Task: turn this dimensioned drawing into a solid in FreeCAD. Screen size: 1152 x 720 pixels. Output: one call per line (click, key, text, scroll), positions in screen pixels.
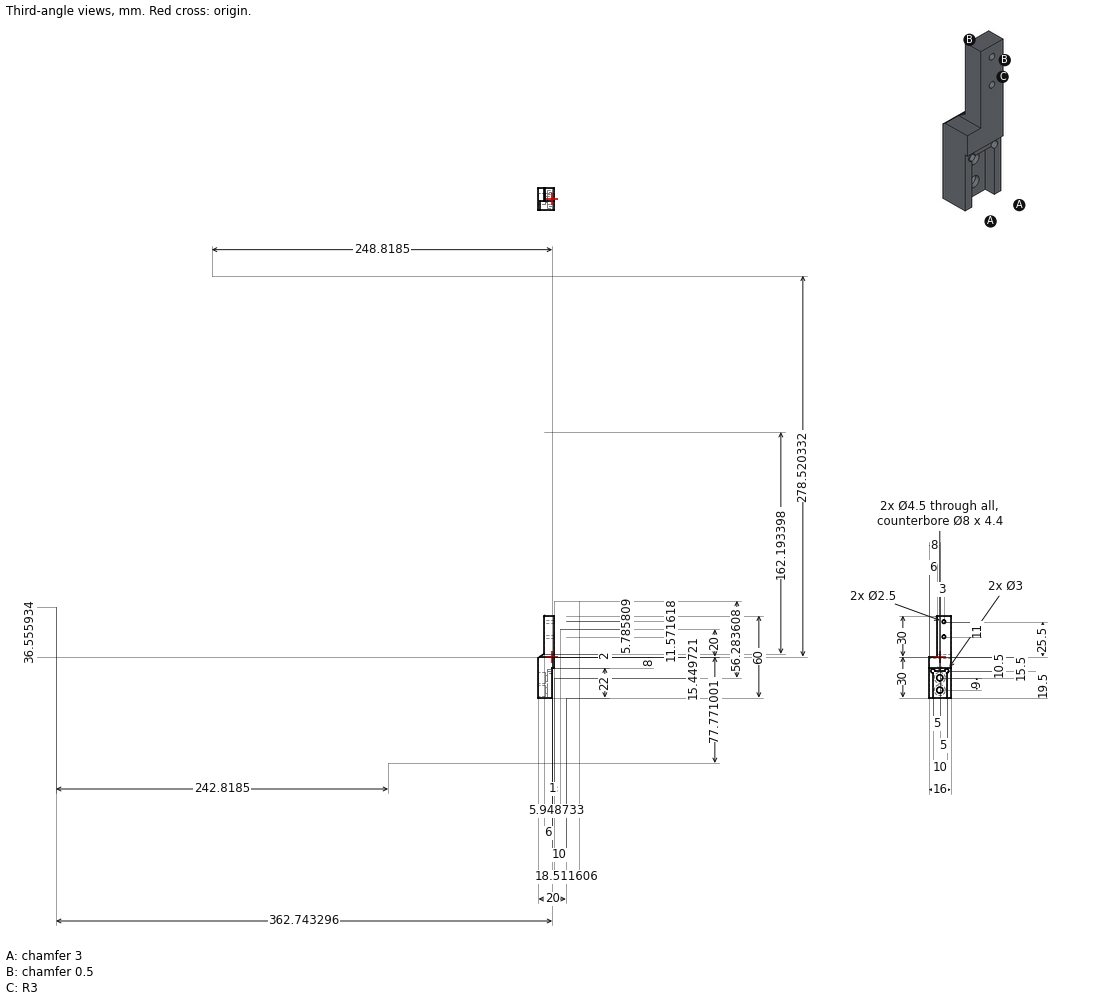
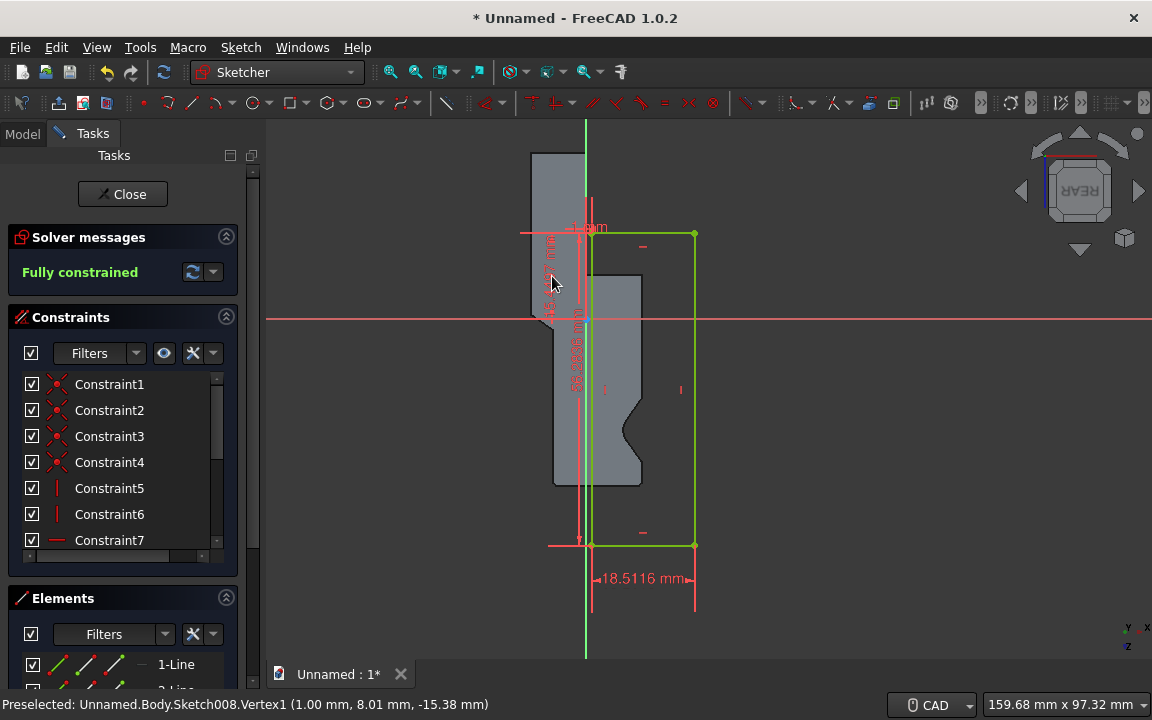
click(123, 194)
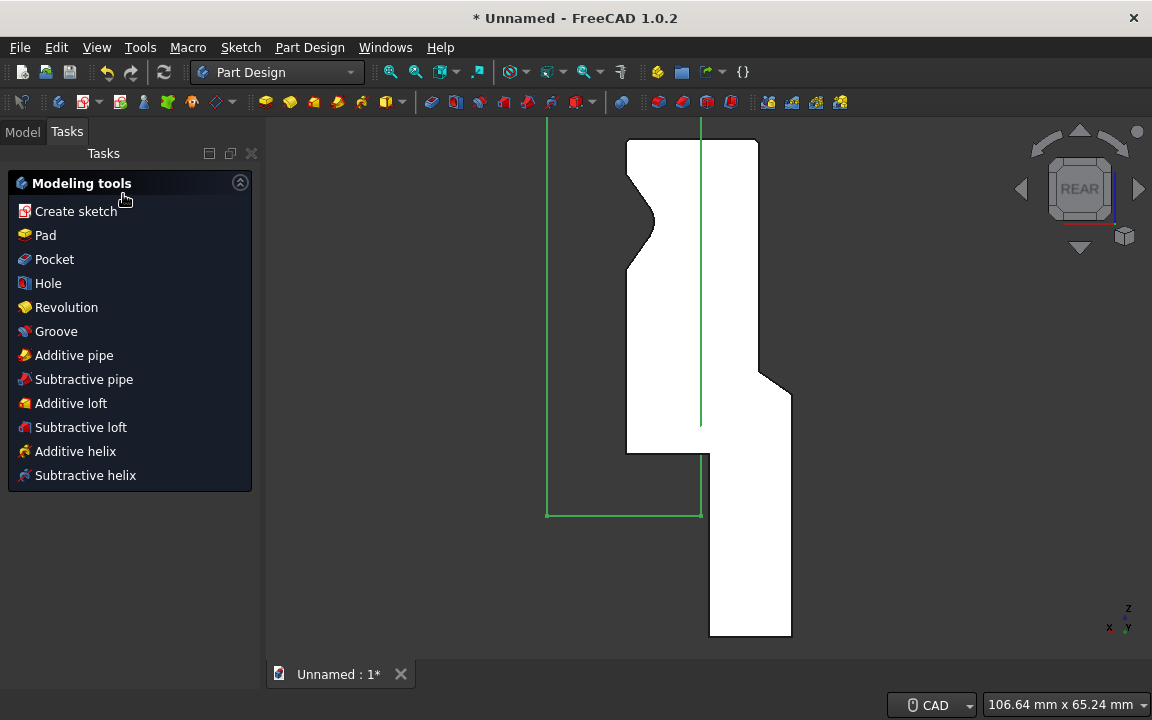
click(432, 102)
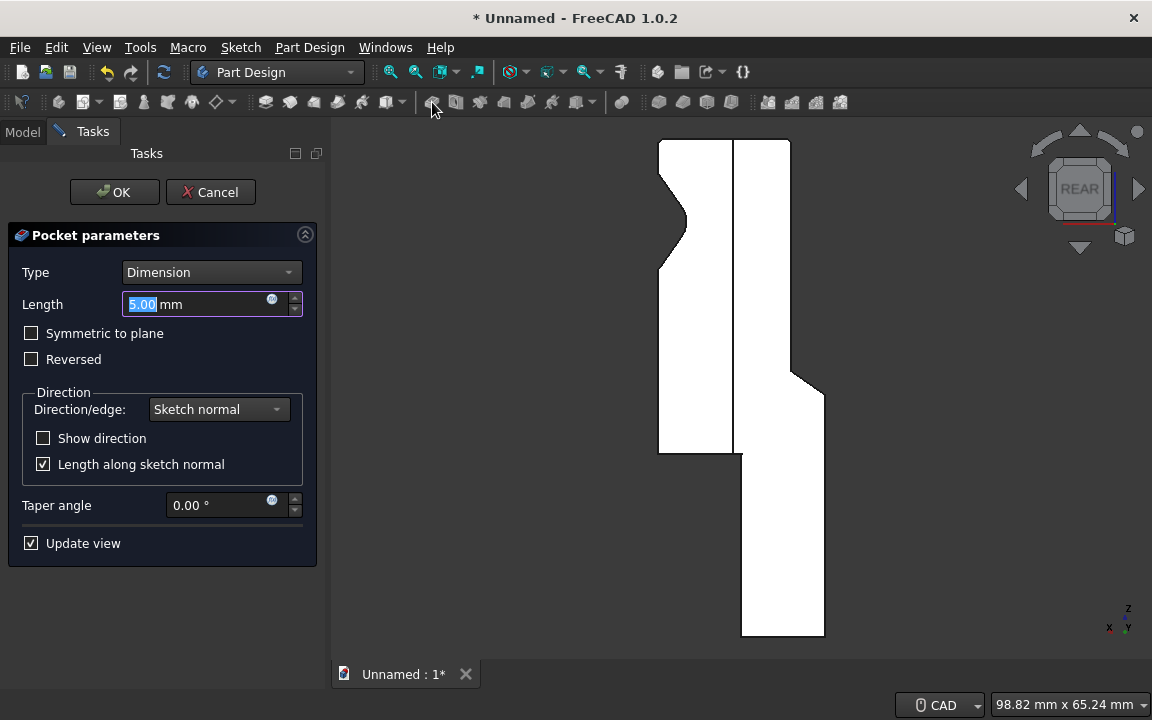
click(212, 272)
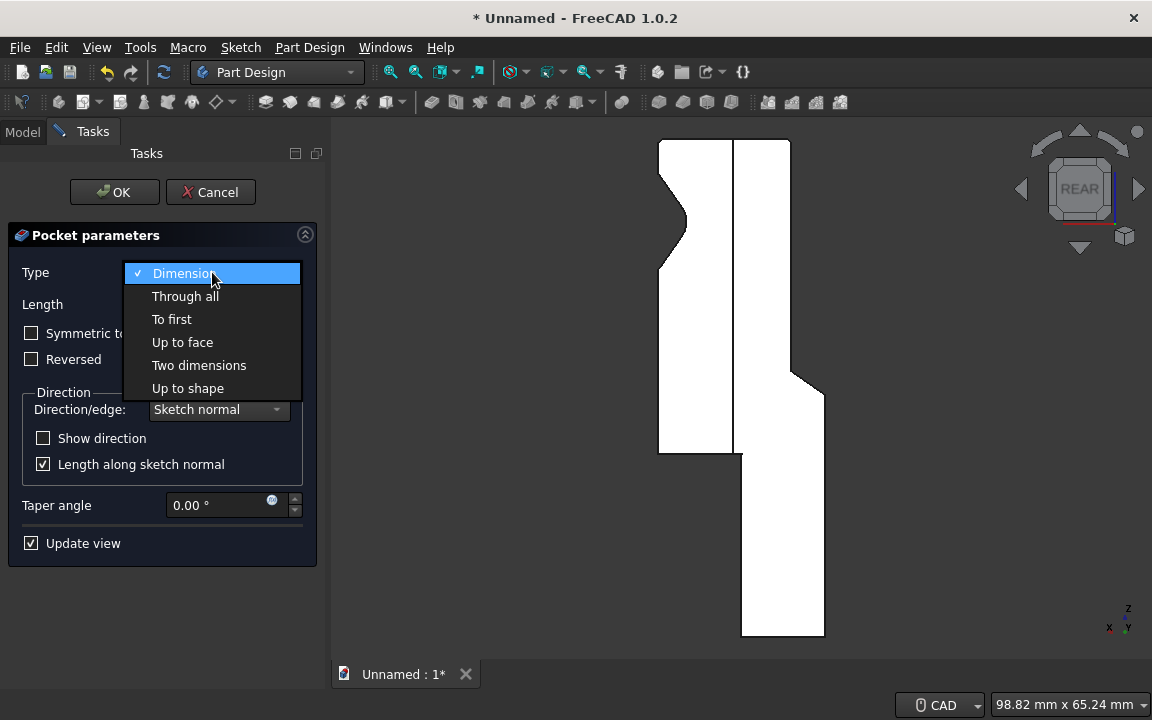
click(212, 296)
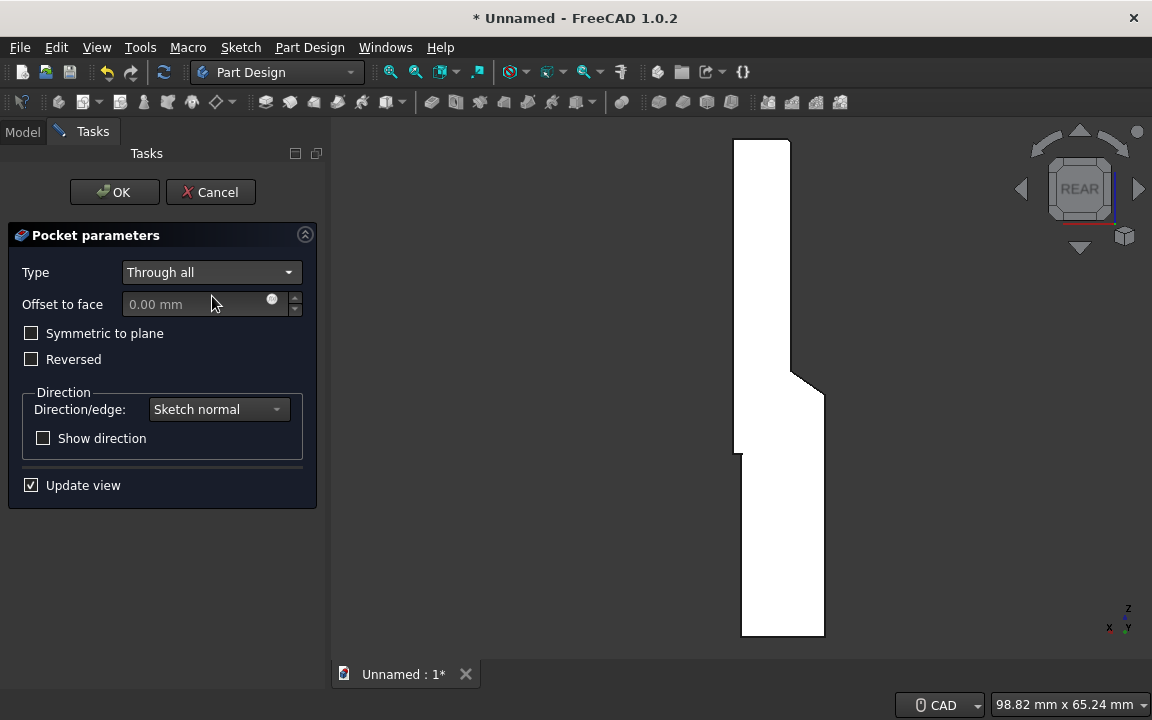
click(115, 192)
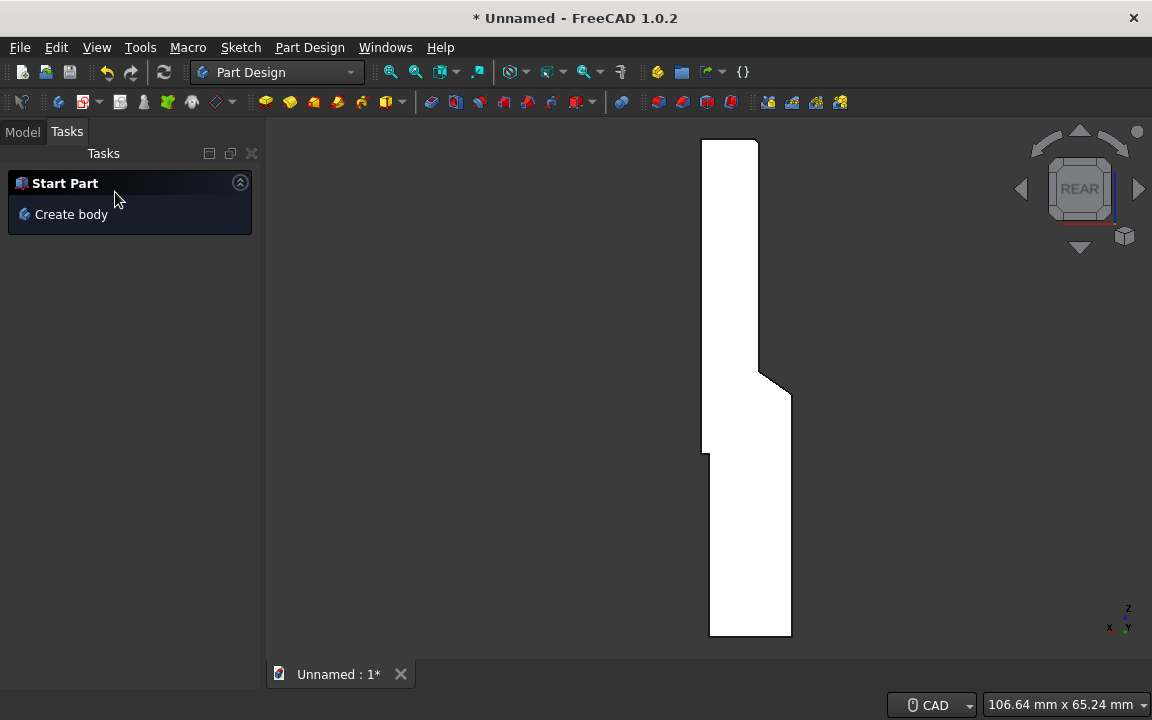
key(0)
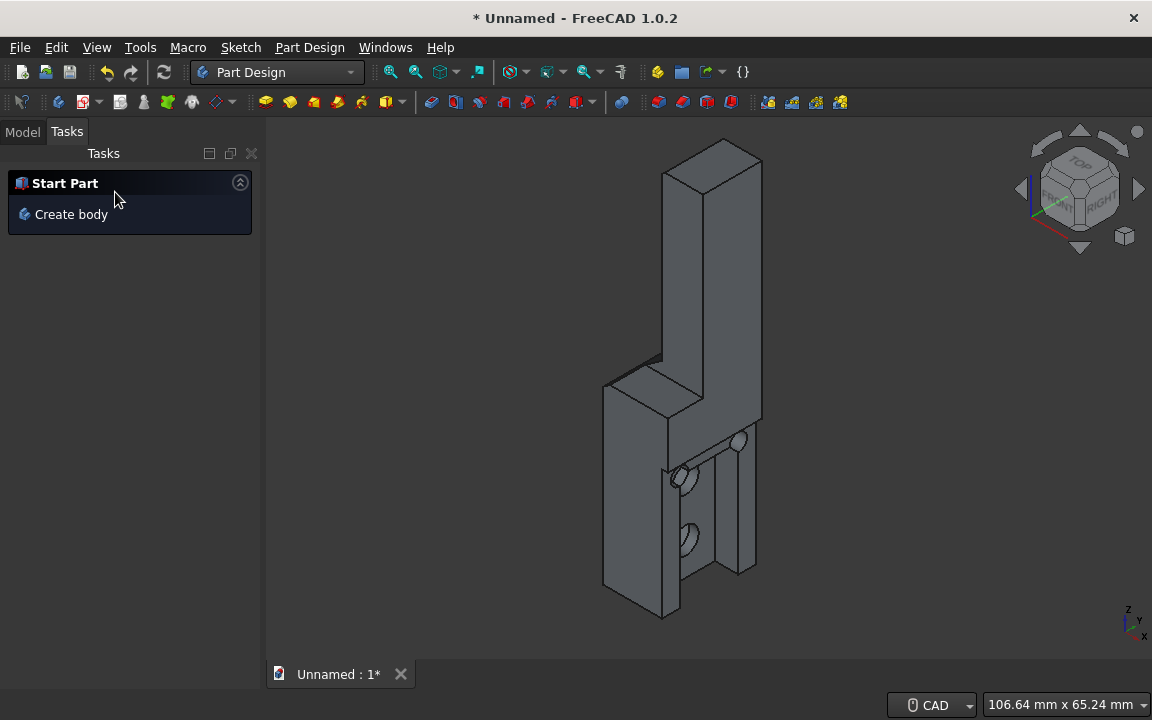
click(728, 382)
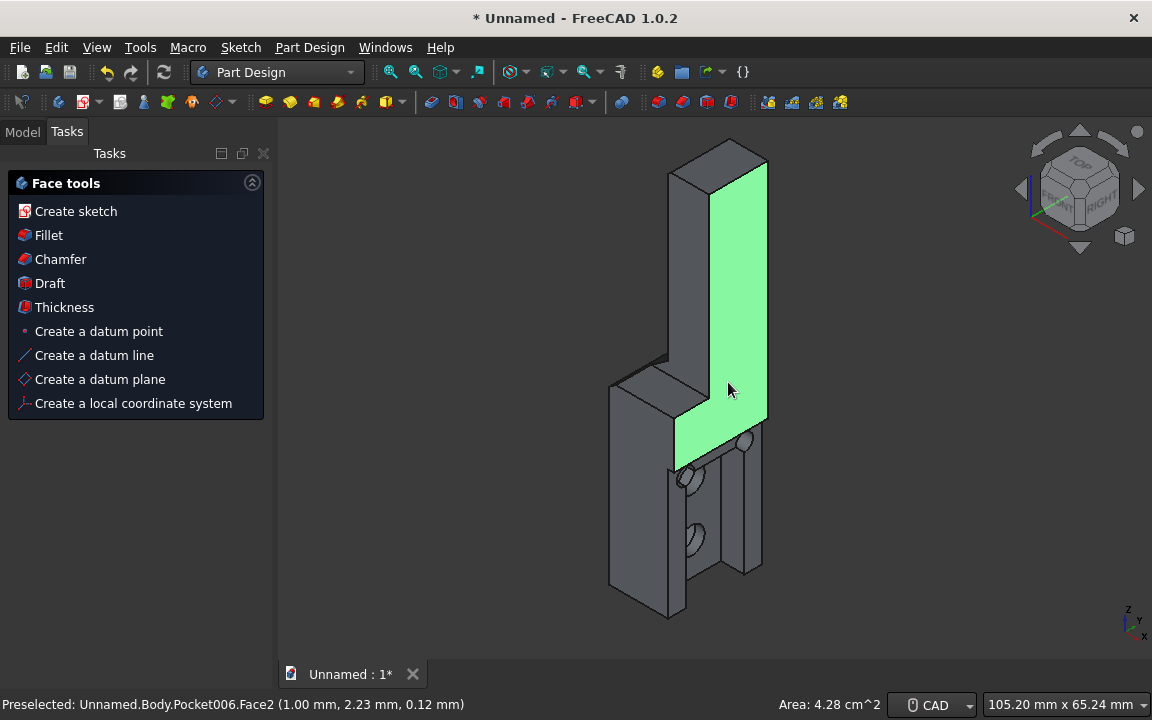
click(84, 102)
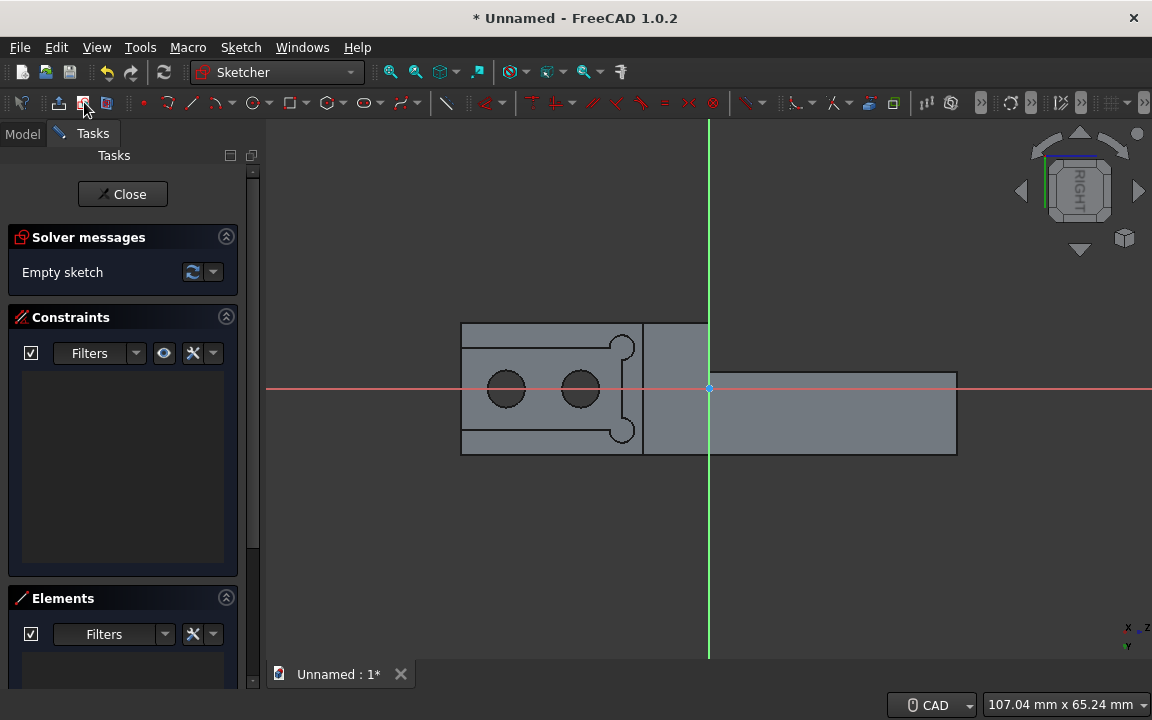
scroll(966, 421, up, 4)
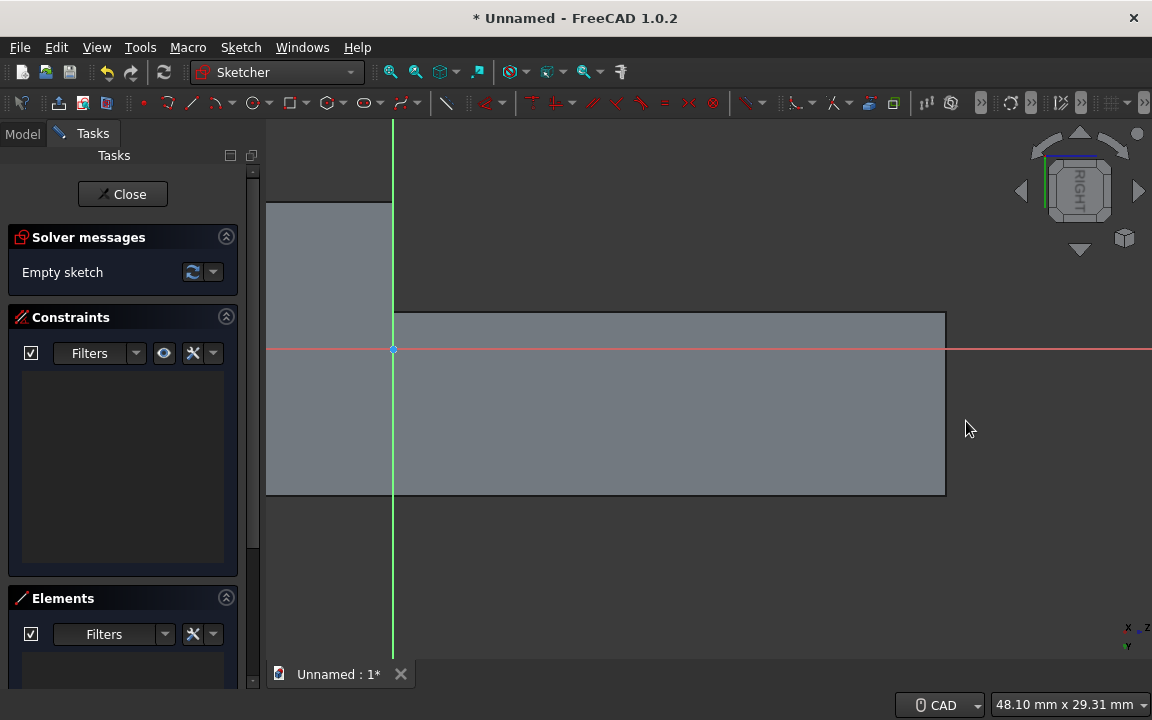
key(g)
key(c)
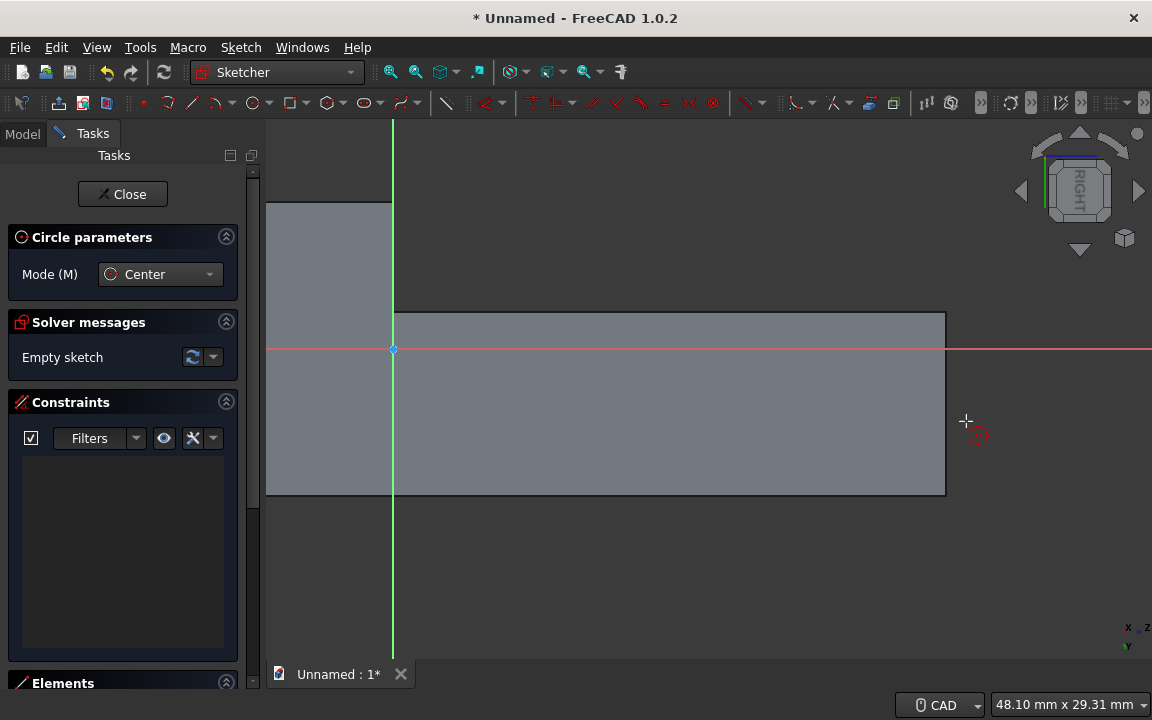
click(863, 404)
click(879, 388)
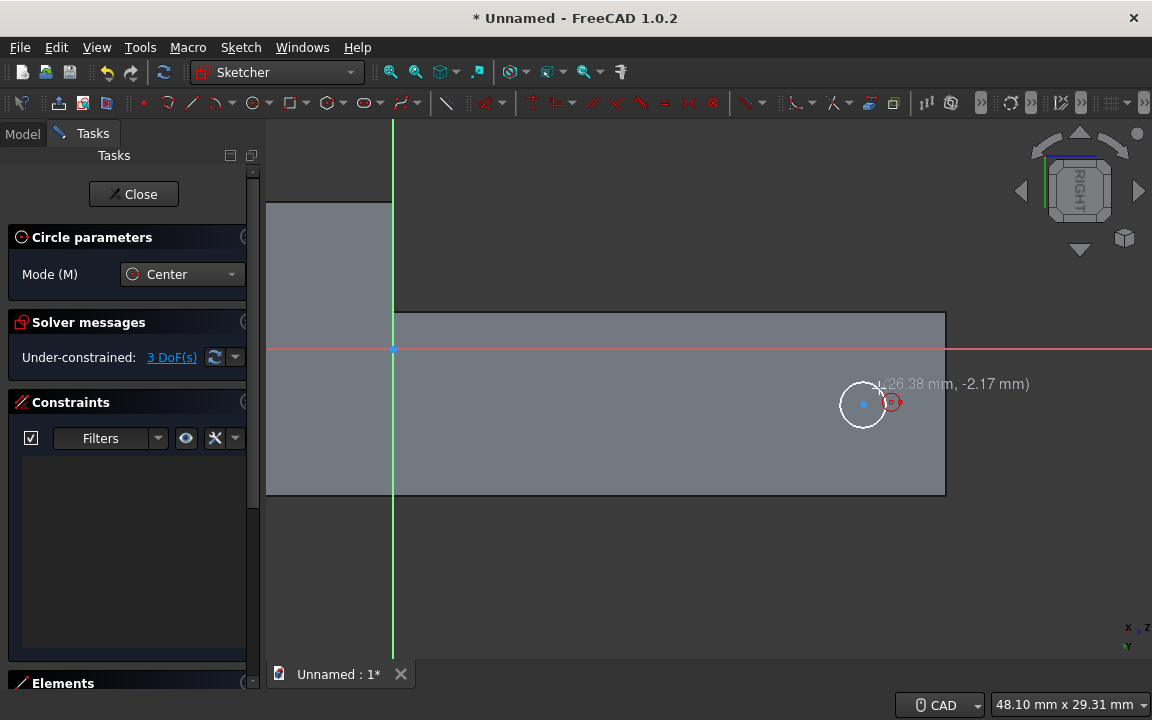
click(660, 404)
click(676, 388)
key(Escape)